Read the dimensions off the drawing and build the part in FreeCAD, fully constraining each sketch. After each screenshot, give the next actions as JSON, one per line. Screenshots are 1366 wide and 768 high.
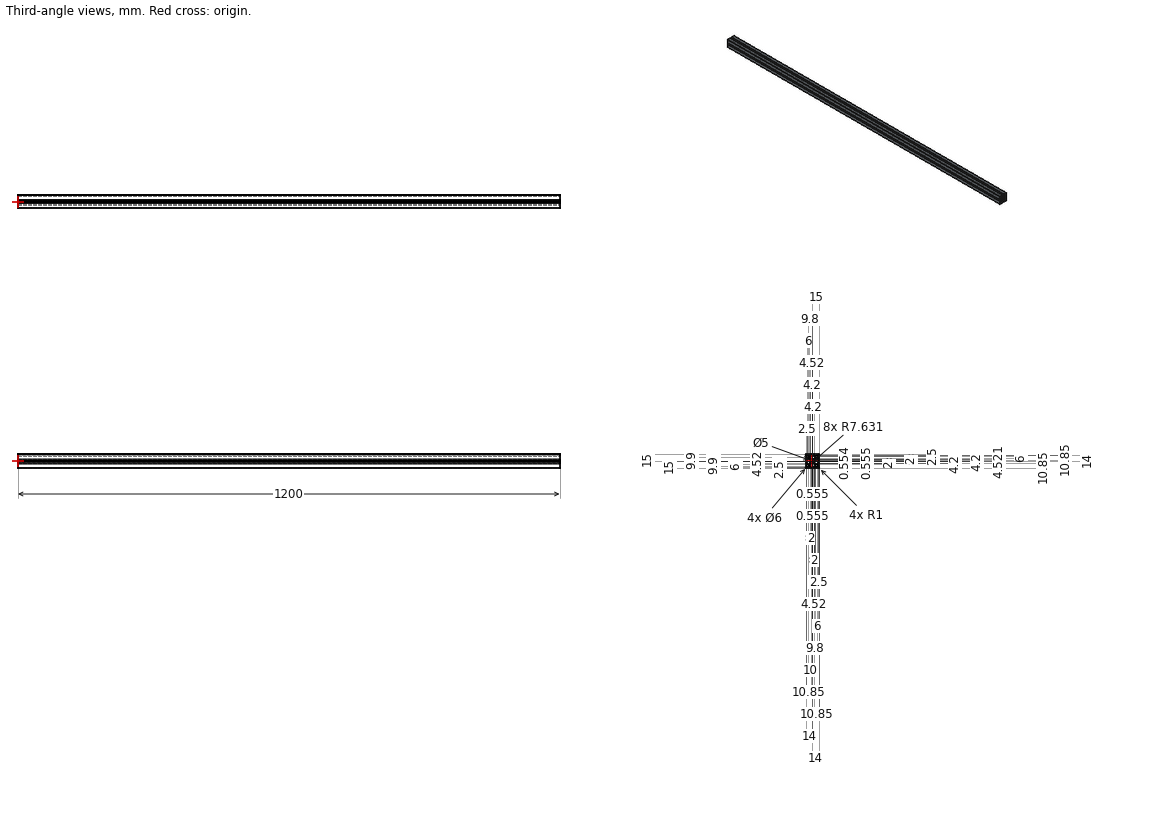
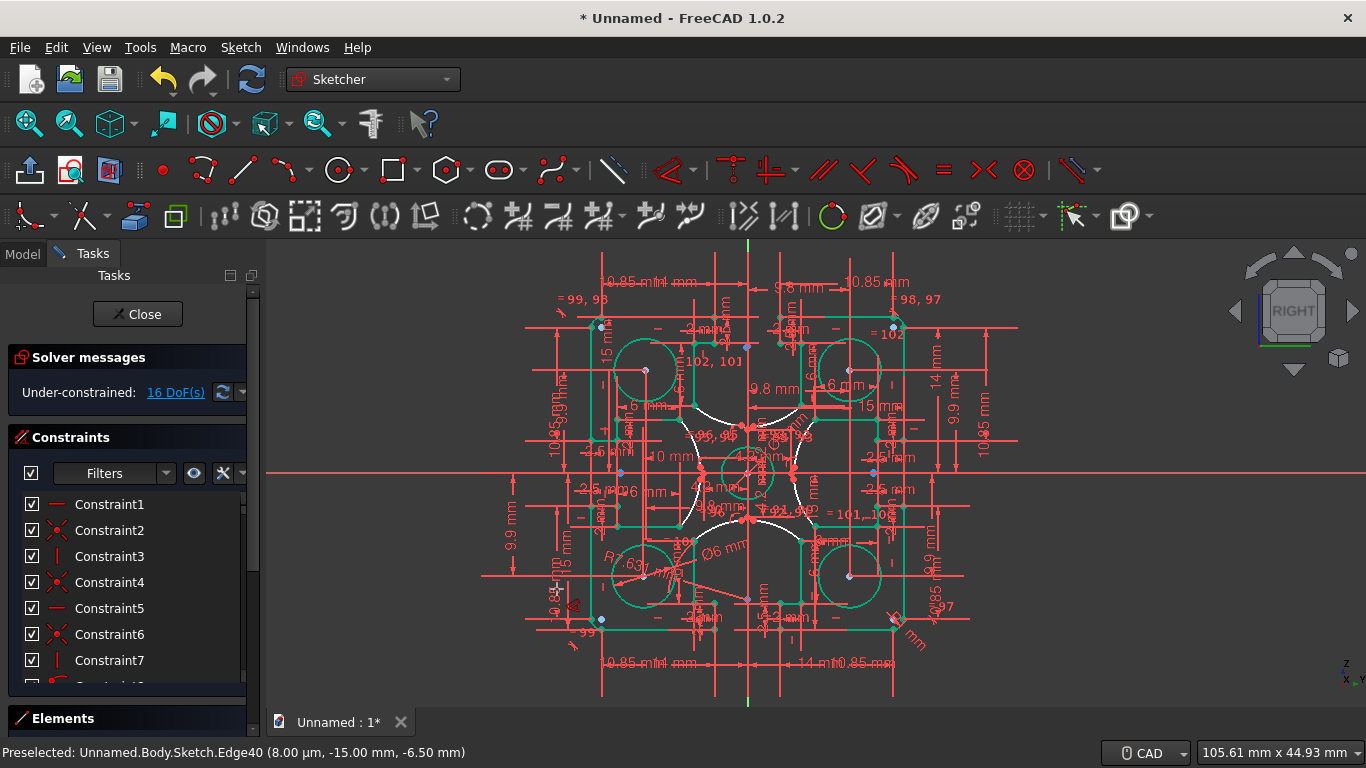
{"action": "scroll", "coordinate": [742, 521], "scroll_direction": "up", "scroll_amount": 3}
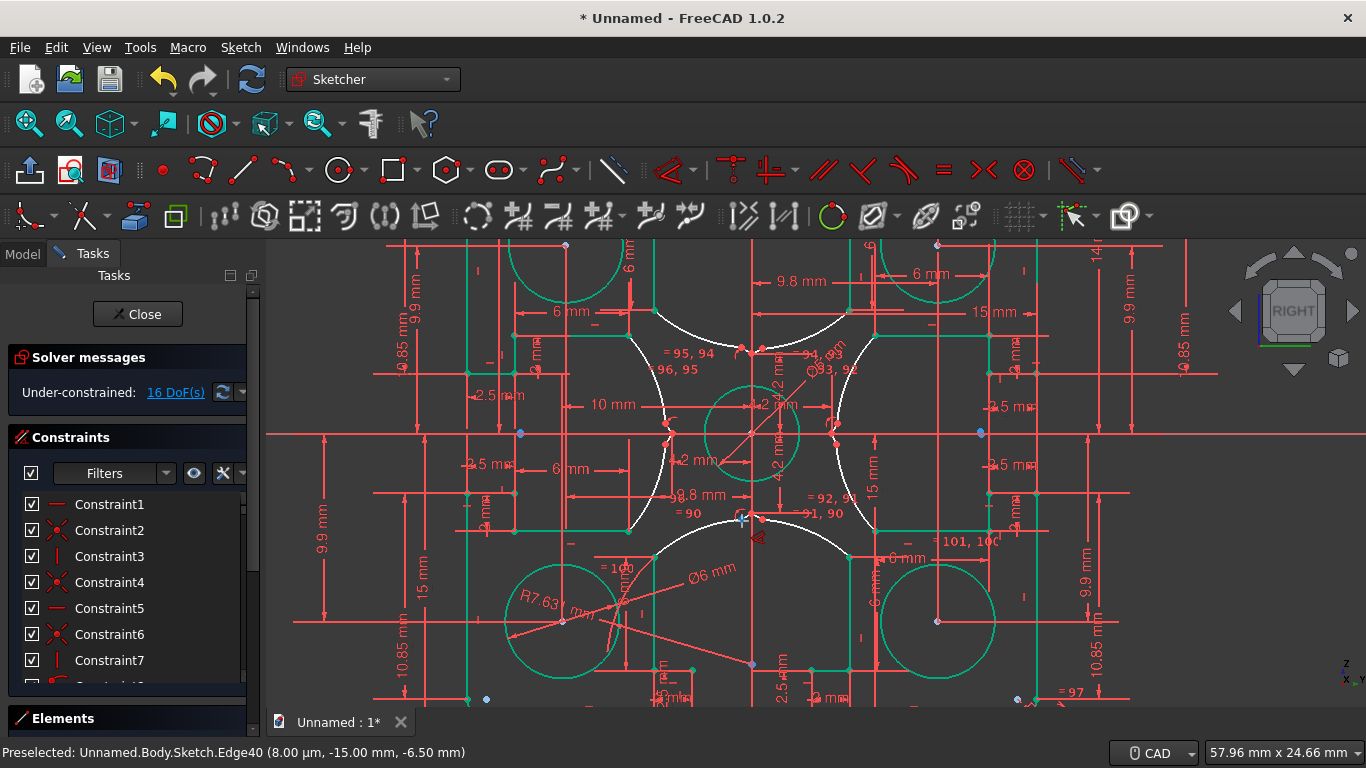
{"action": "left_click", "coordinate": [741, 520]}
{"action": "left_click", "coordinate": [786, 497]}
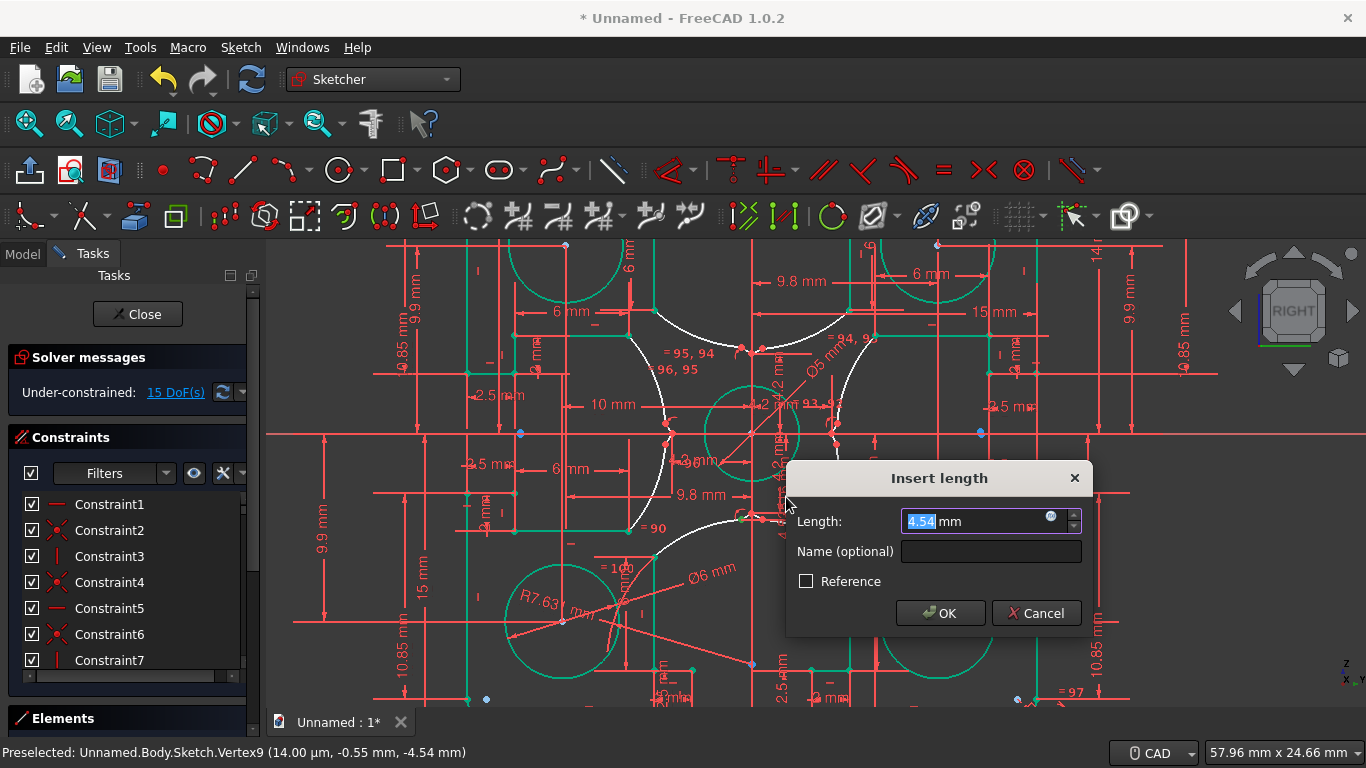
{"action": "type", "text": "4.52"}
{"action": "key", "text": "Return"}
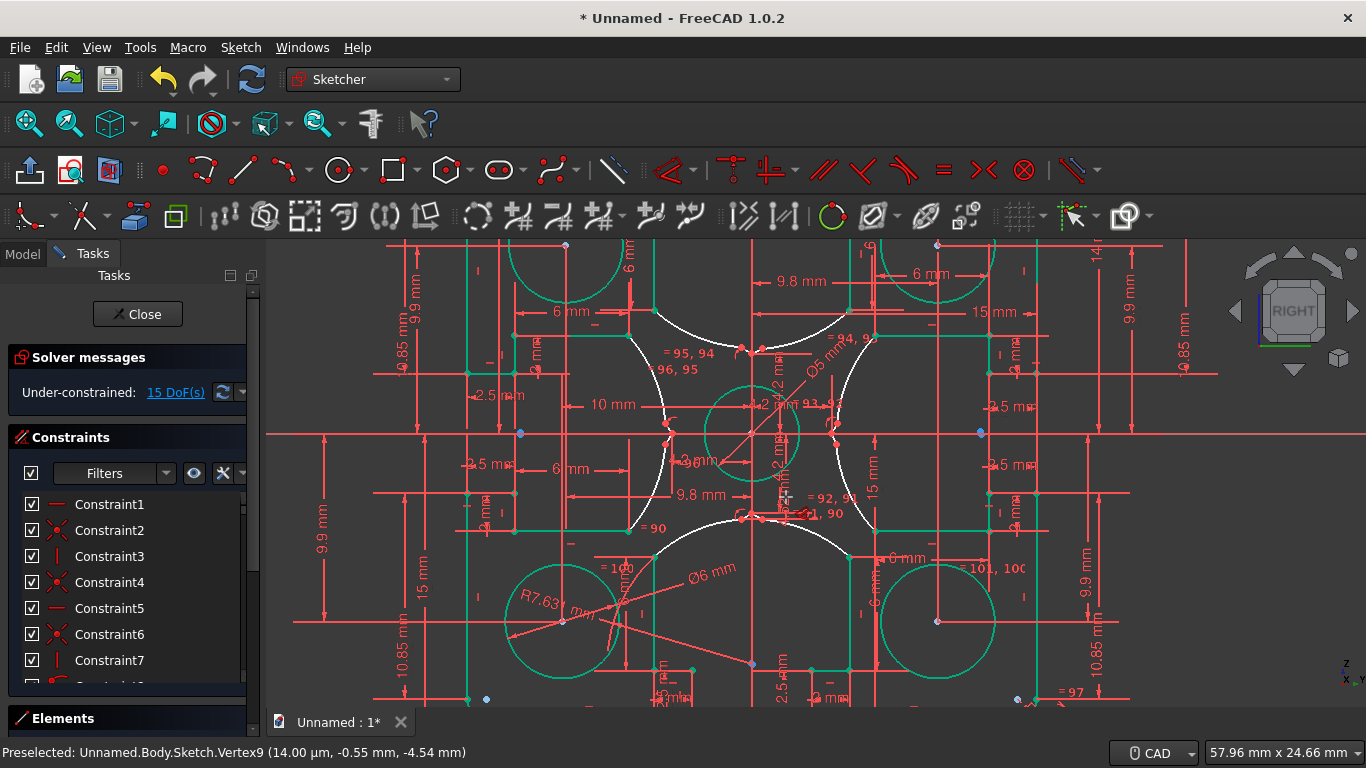
{"action": "left_click", "coordinate": [762, 520]}
{"action": "left_click", "coordinate": [868, 497]}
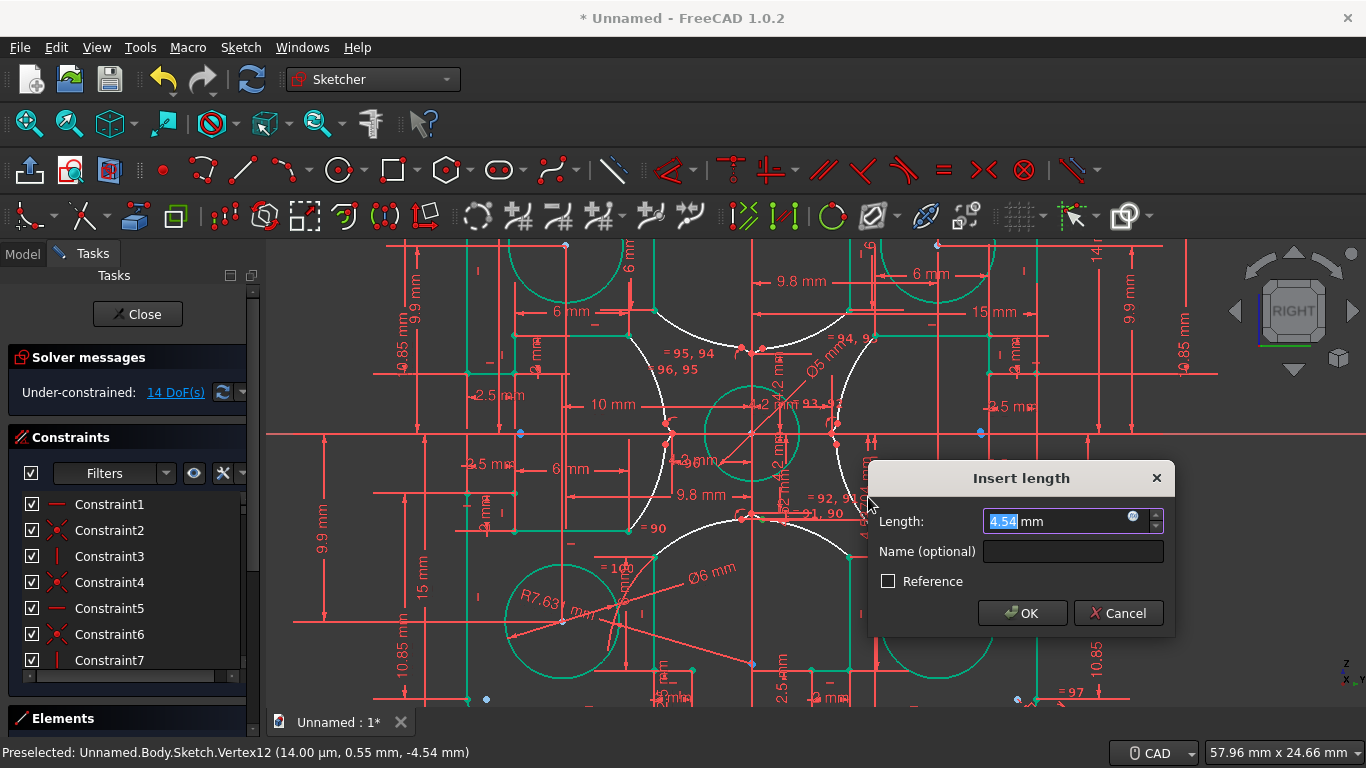
{"action": "type", "text": "4.52"}
{"action": "key", "text": "Return"}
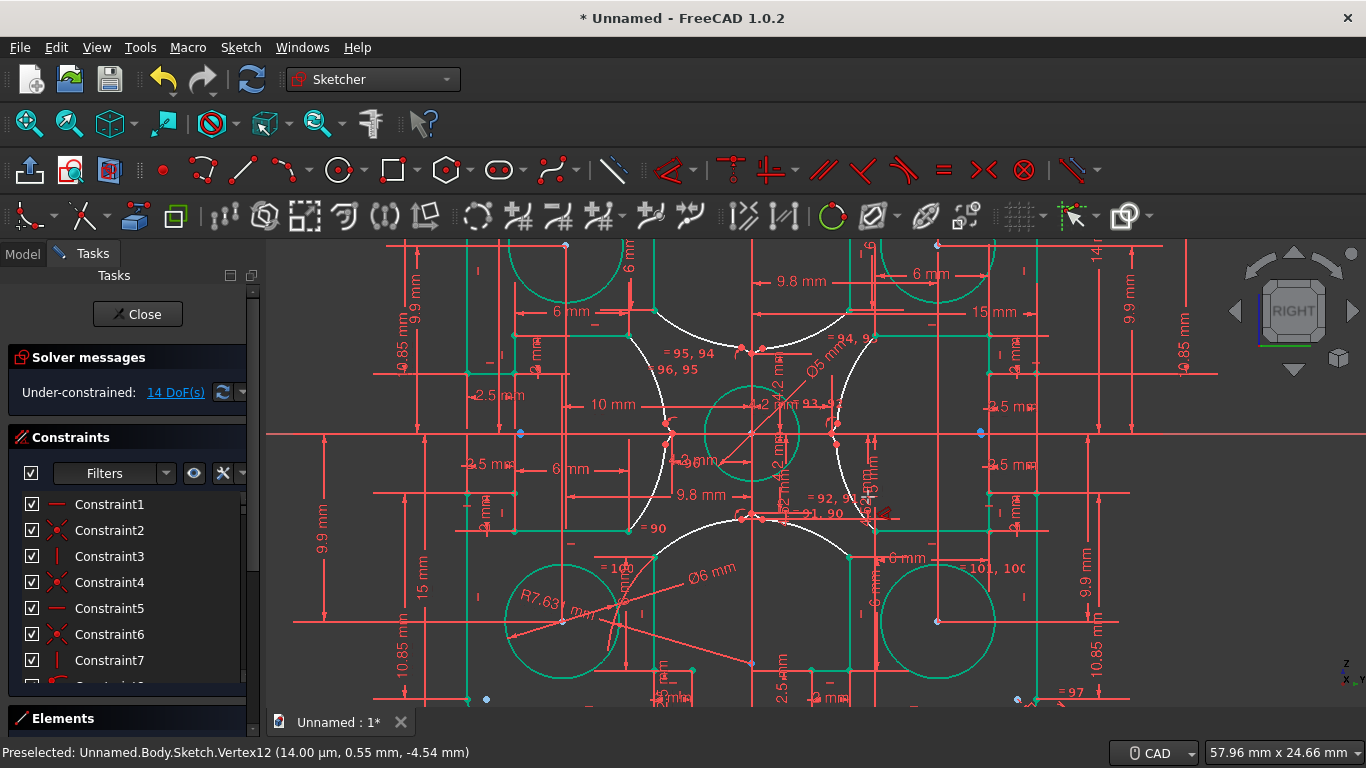
{"action": "left_click", "coordinate": [836, 444]}
{"action": "left_click", "coordinate": [794, 550]}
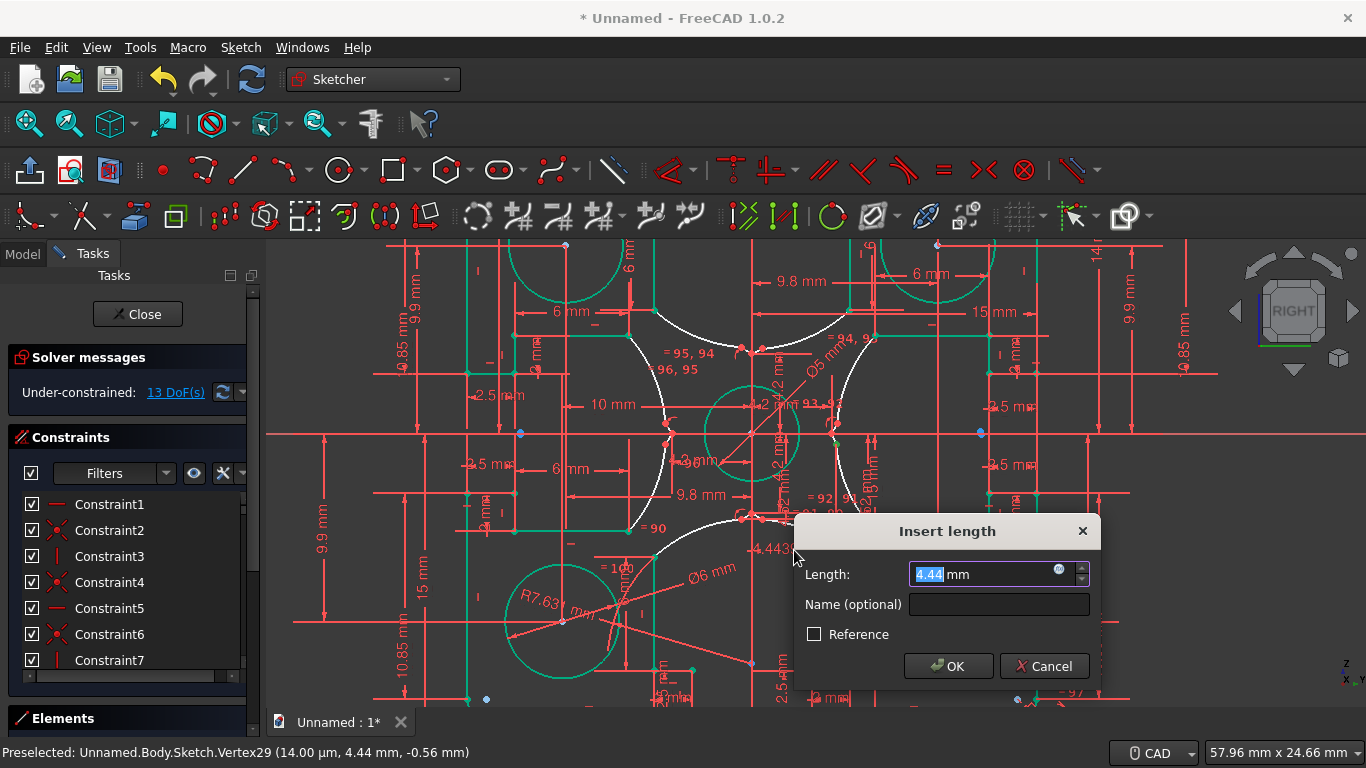
{"action": "type", "text": "4.52"}
{"action": "key", "text": "Return"}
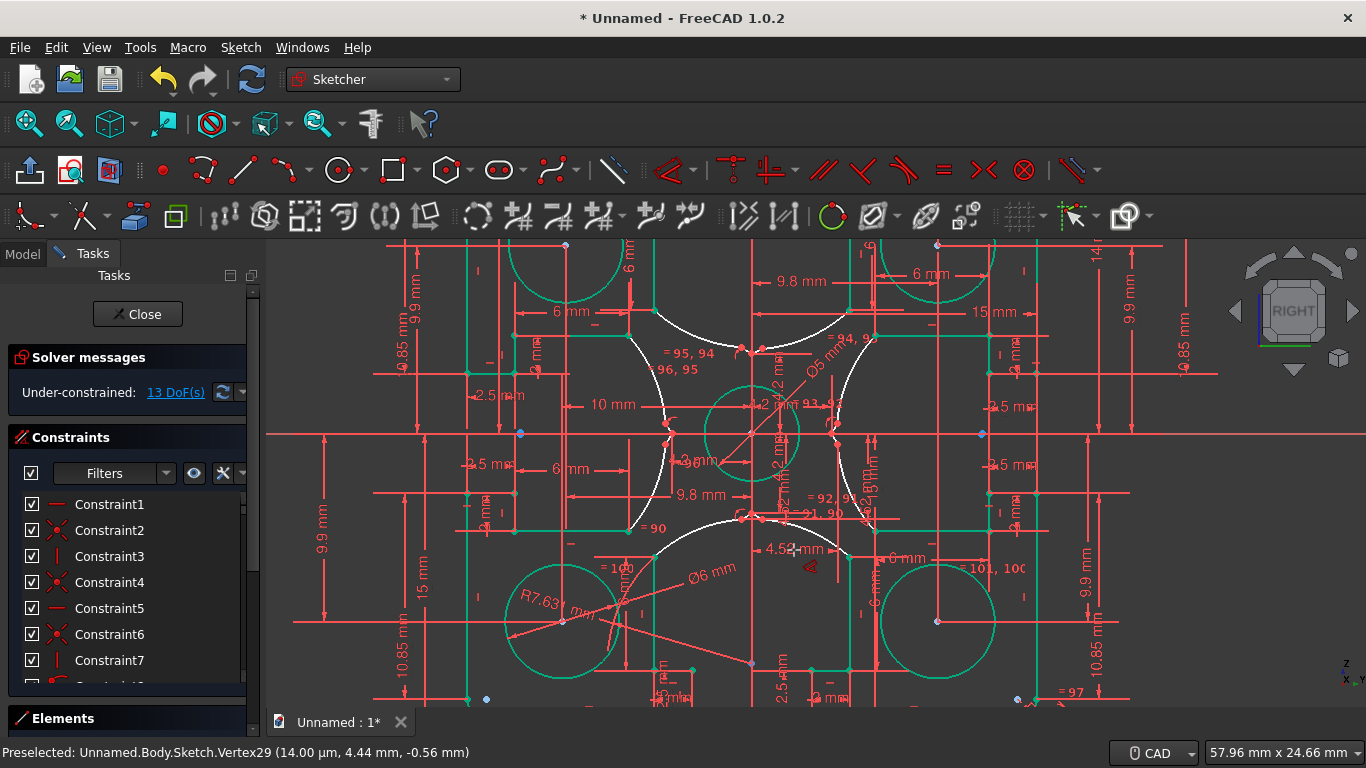
{"action": "left_click", "coordinate": [837, 424]}
{"action": "left_click", "coordinate": [795, 318]}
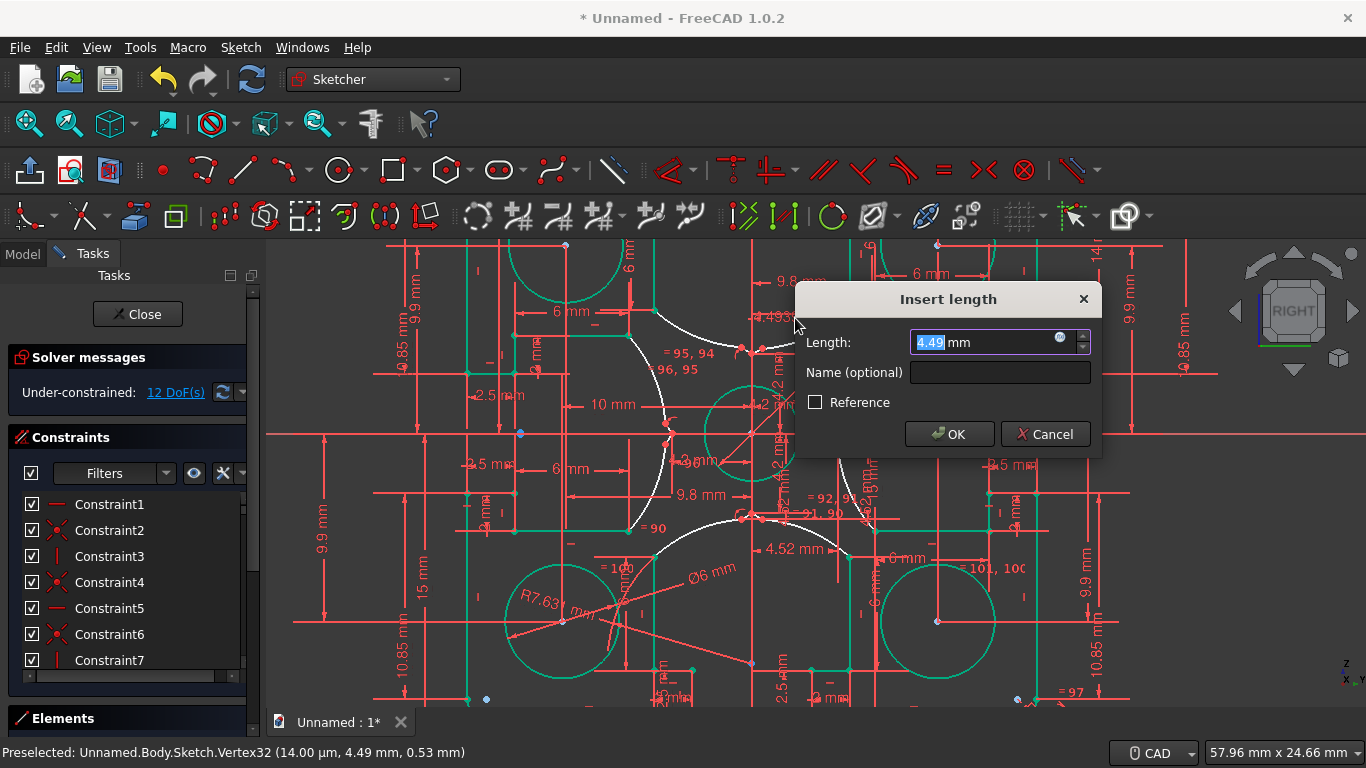
{"action": "type", "text": "4.52"}
{"action": "key", "text": "Return"}